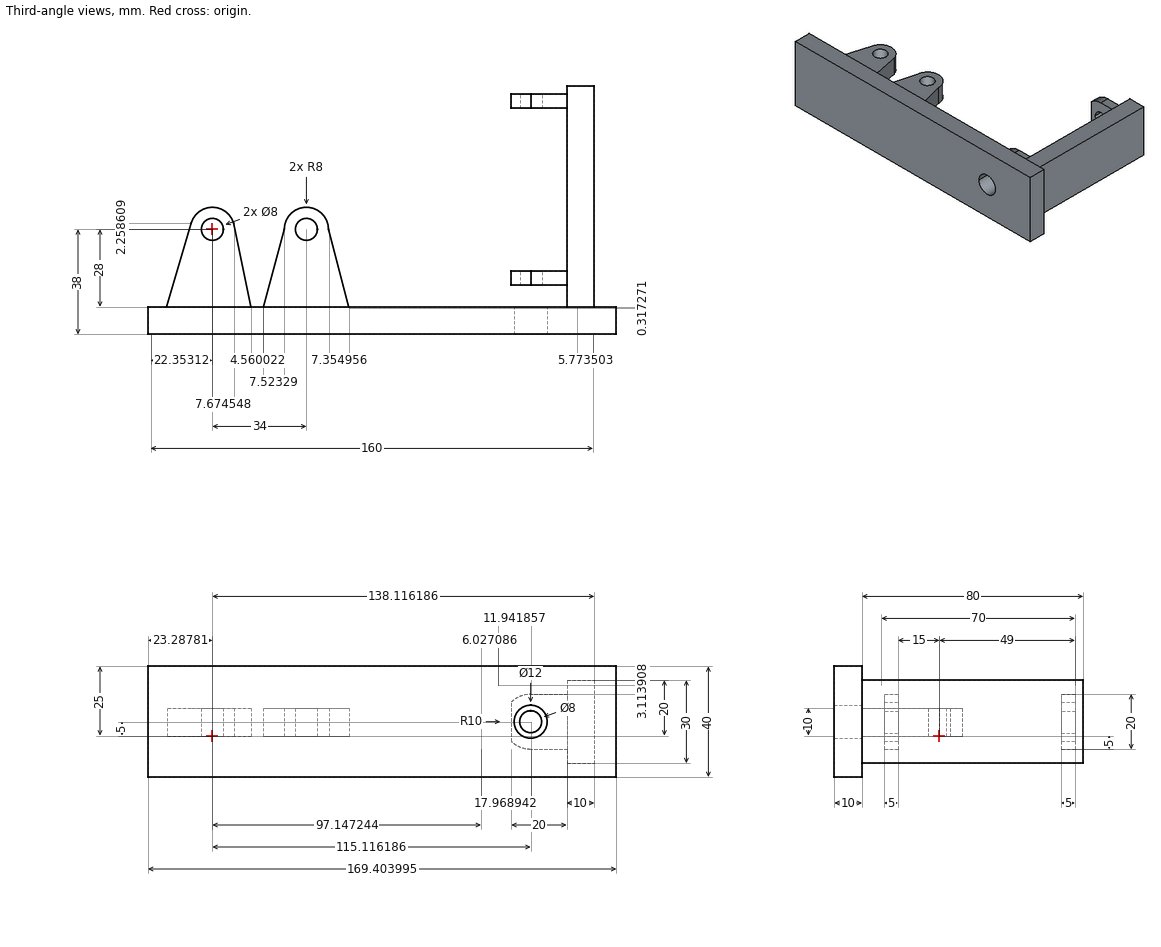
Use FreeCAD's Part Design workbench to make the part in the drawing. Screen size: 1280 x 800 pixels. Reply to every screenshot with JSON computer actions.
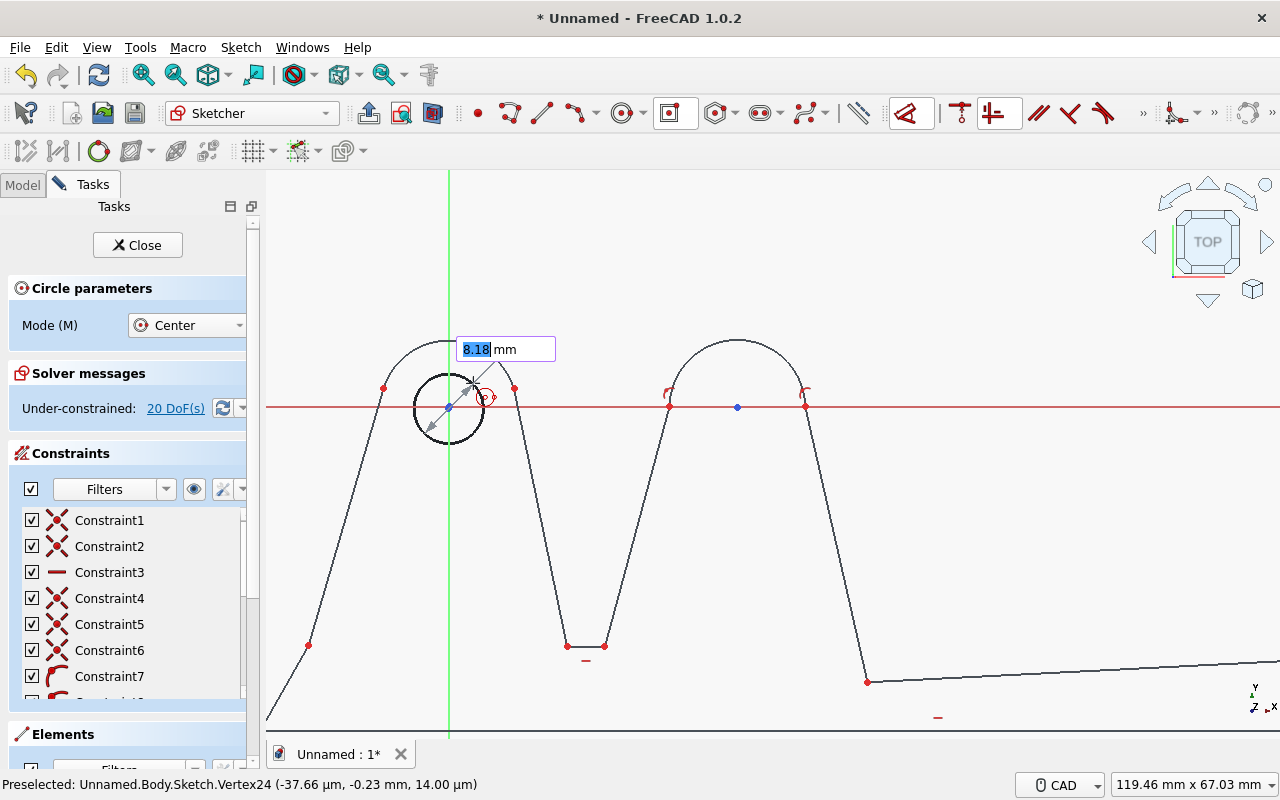
{"action": "type", "text": "8"}
{"action": "key", "text": "Return"}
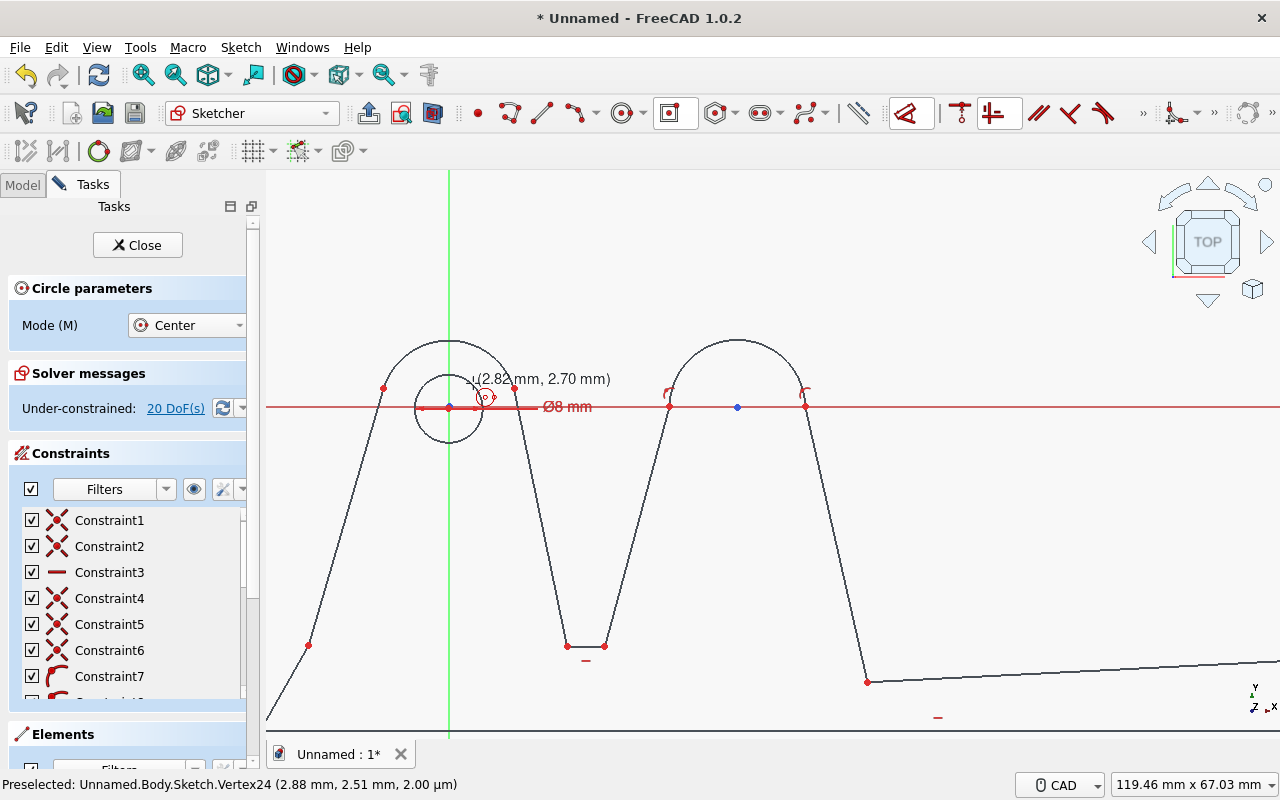
{"action": "left_click", "coordinate": [738, 407]}
{"action": "mouse_move", "coordinate": [762, 383]}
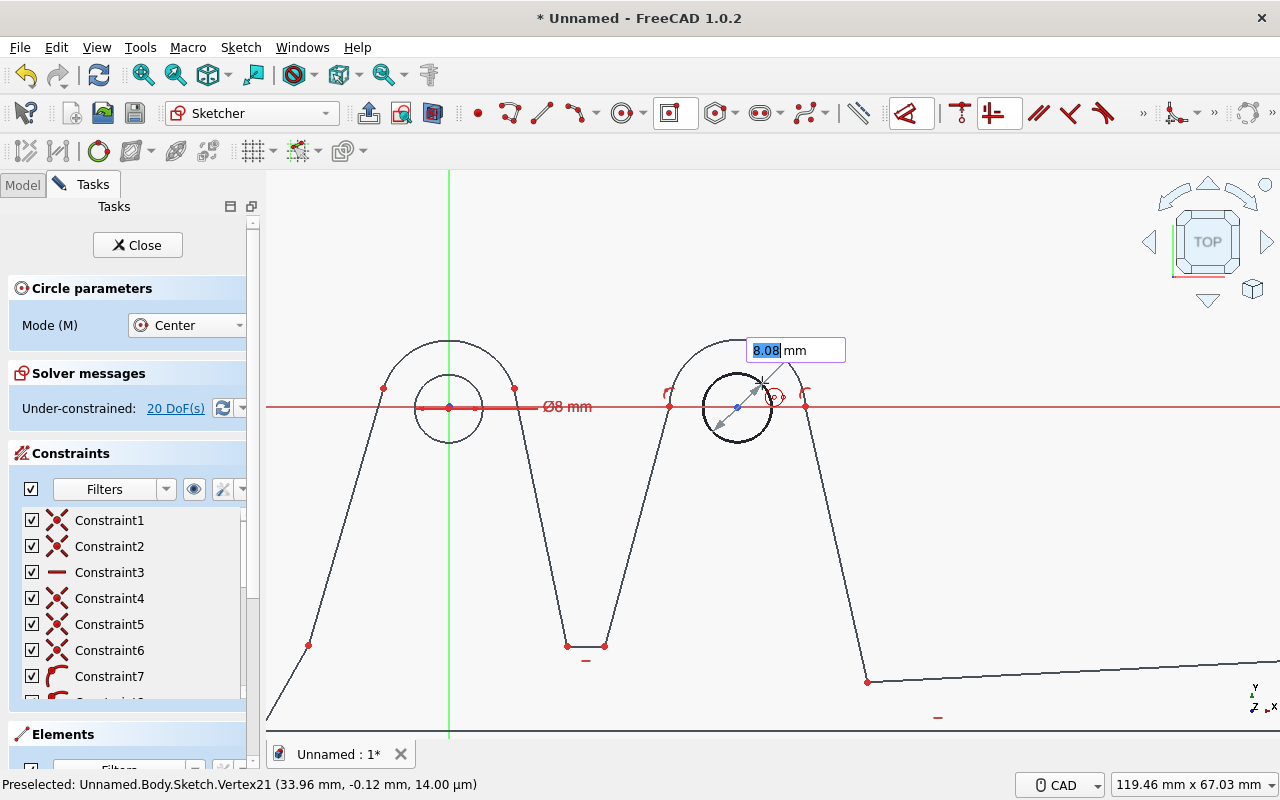
{"action": "type", "text": "8"}
{"action": "key", "text": "Return"}
{"action": "key", "text": "Escape"}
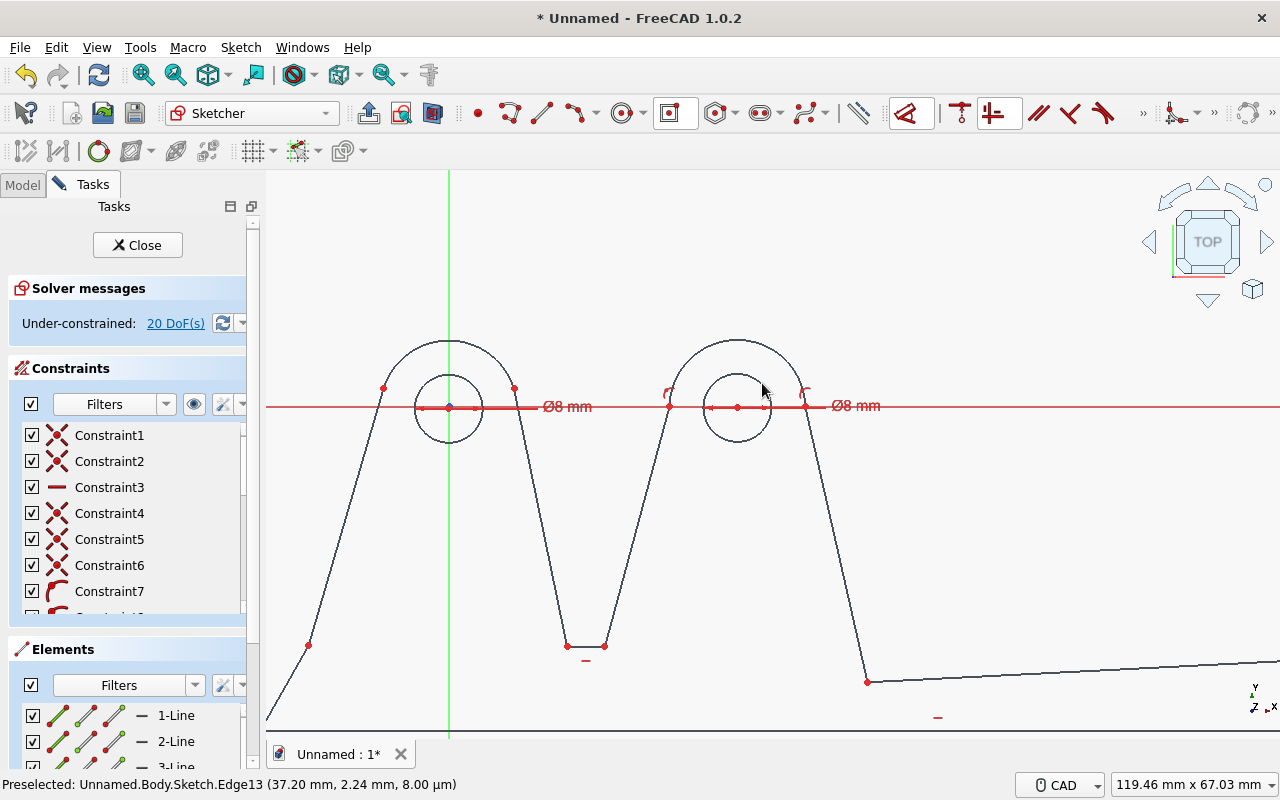
{"action": "left_click", "coordinate": [361, 466]}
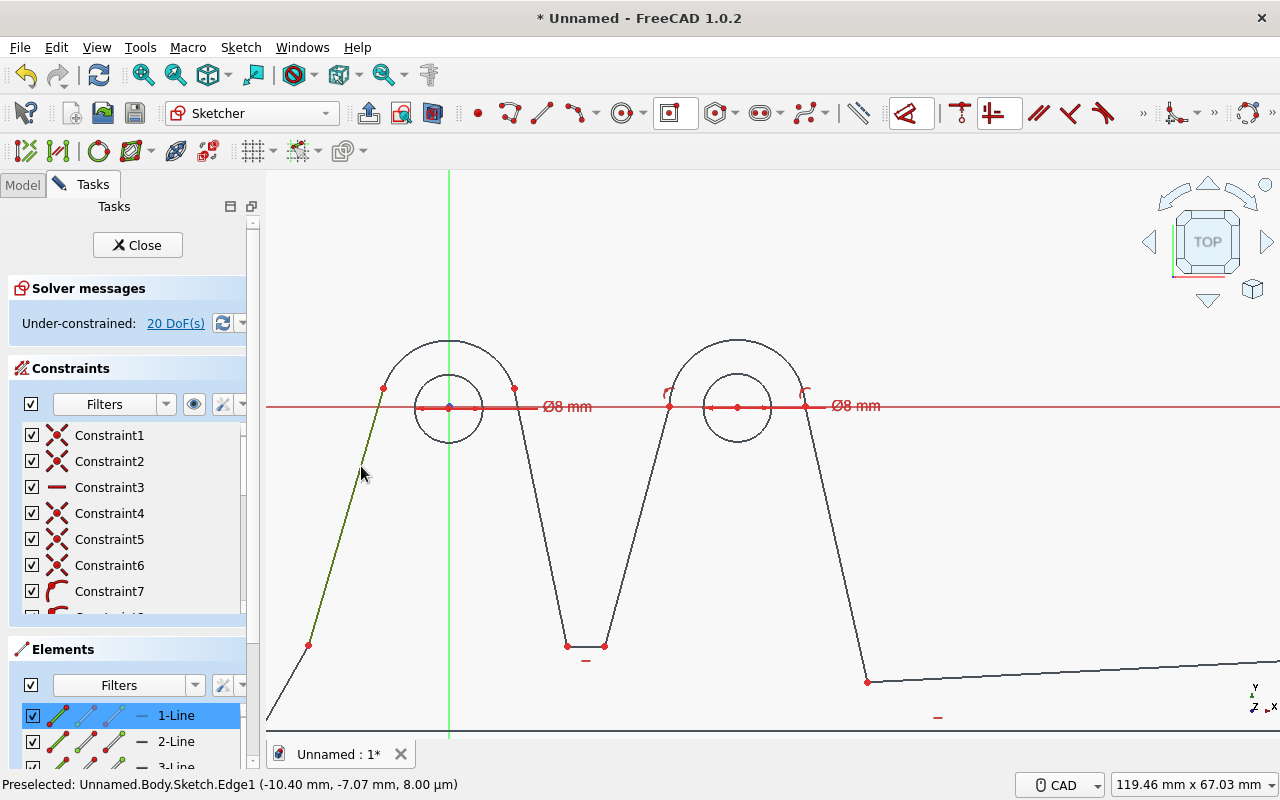
{"action": "left_click", "coordinate": [482, 349]}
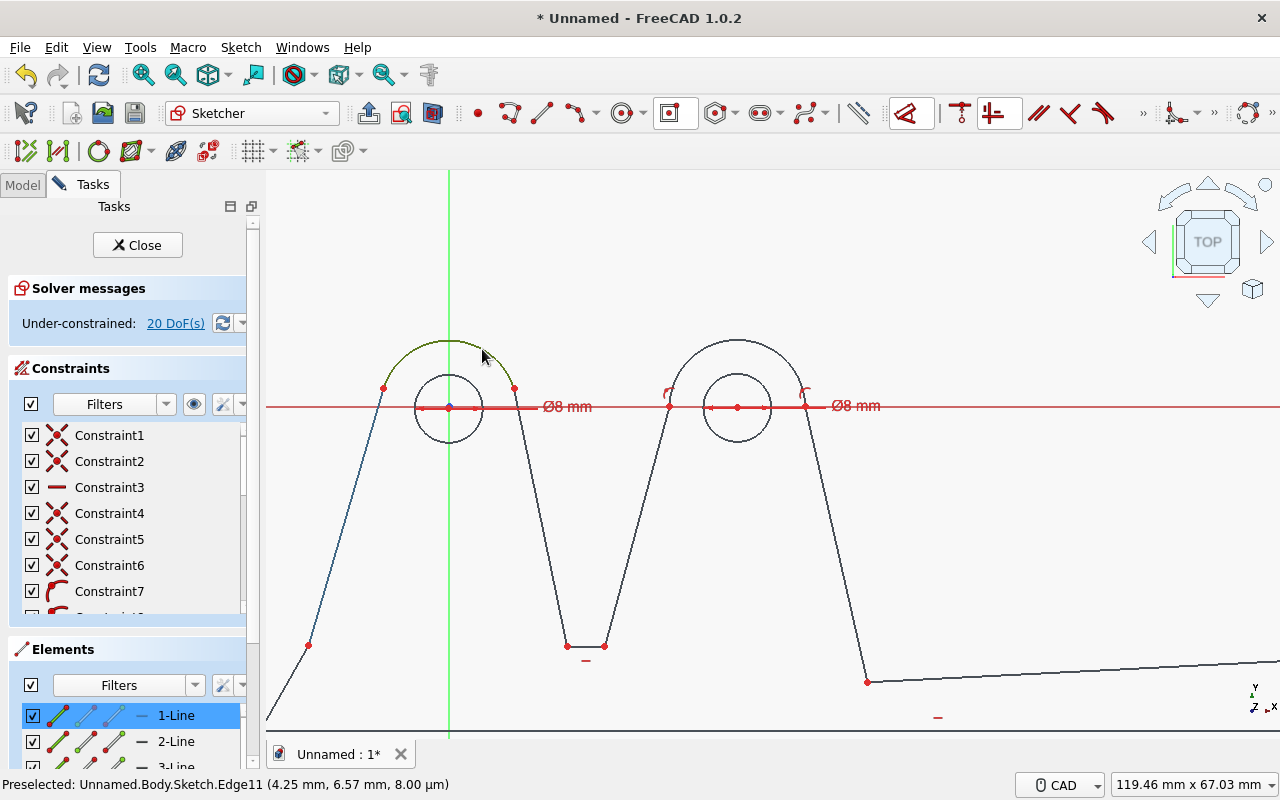
{"action": "left_click", "coordinate": [1104, 114]}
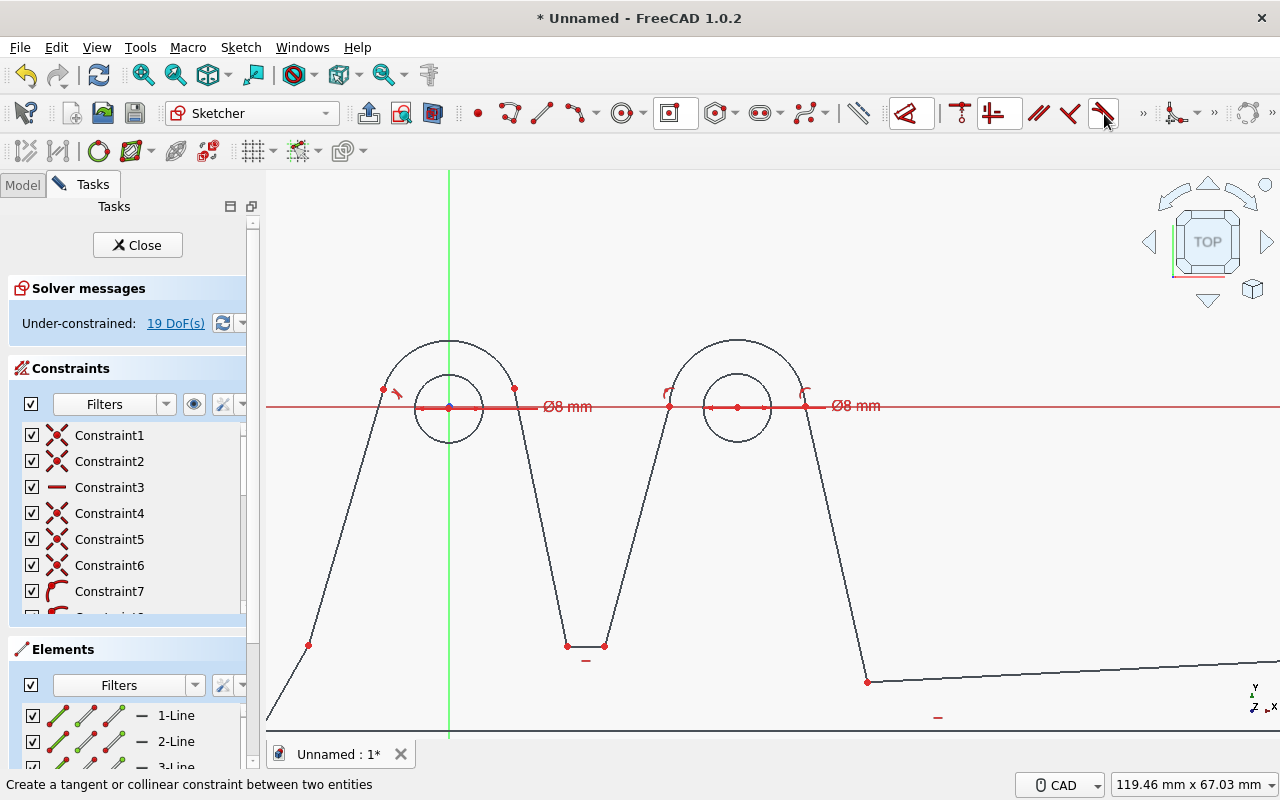
{"action": "left_click_drag", "start_coordinate": [439, 397], "coordinate": [459, 419]}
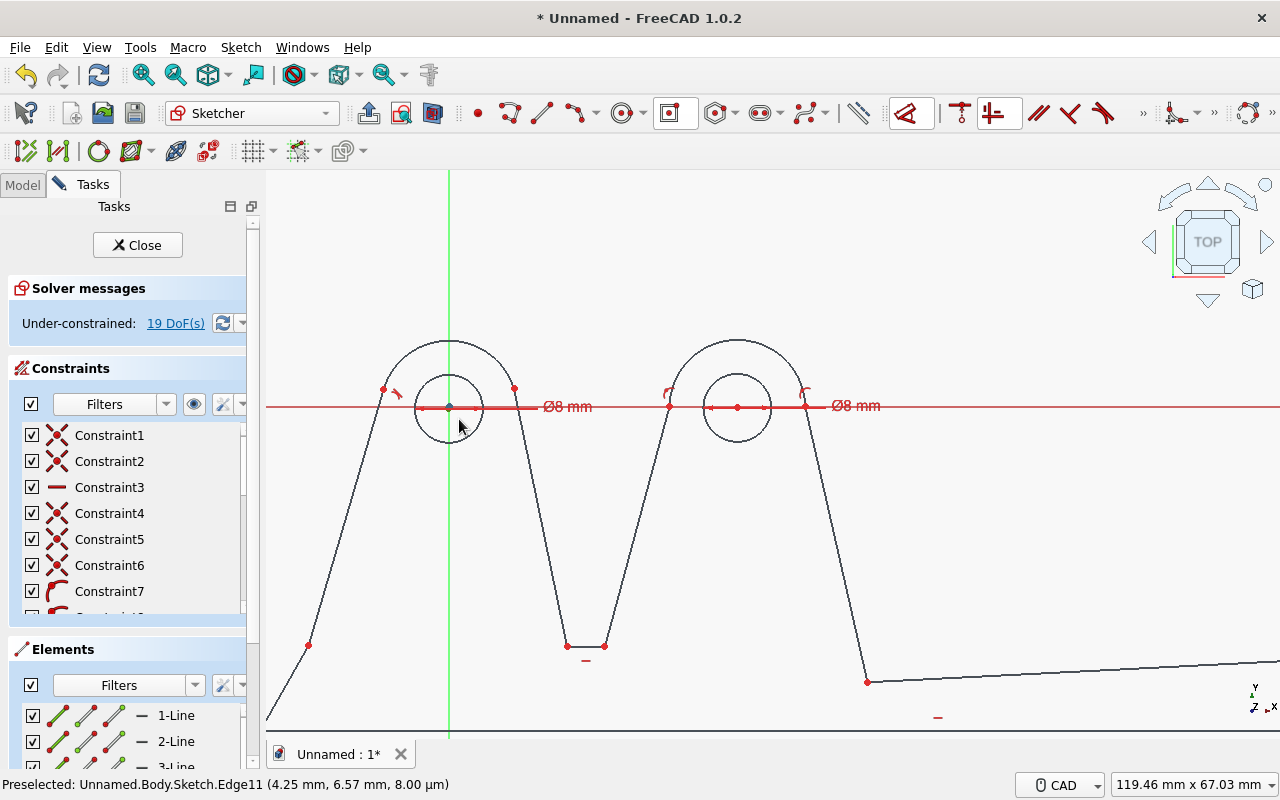
{"action": "left_click", "coordinate": [960, 114]}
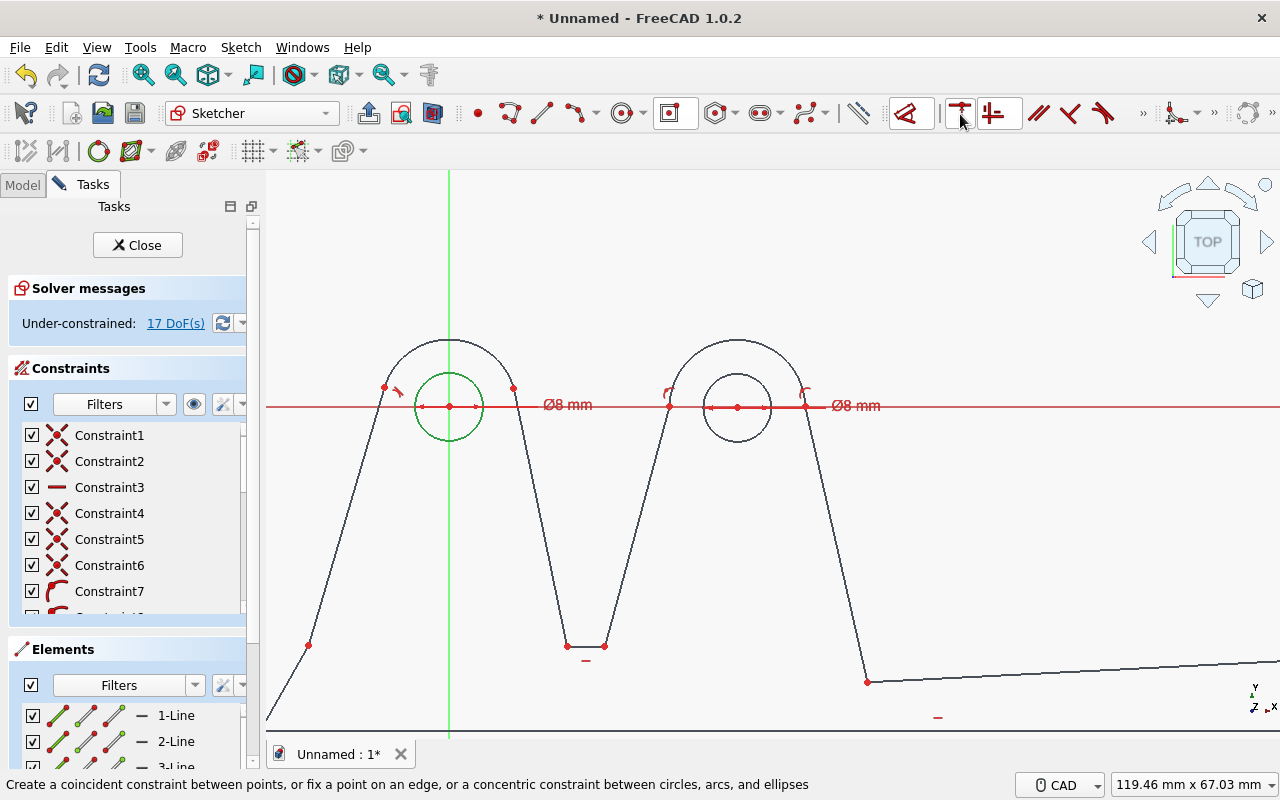
{"action": "left_click", "coordinate": [777, 353]}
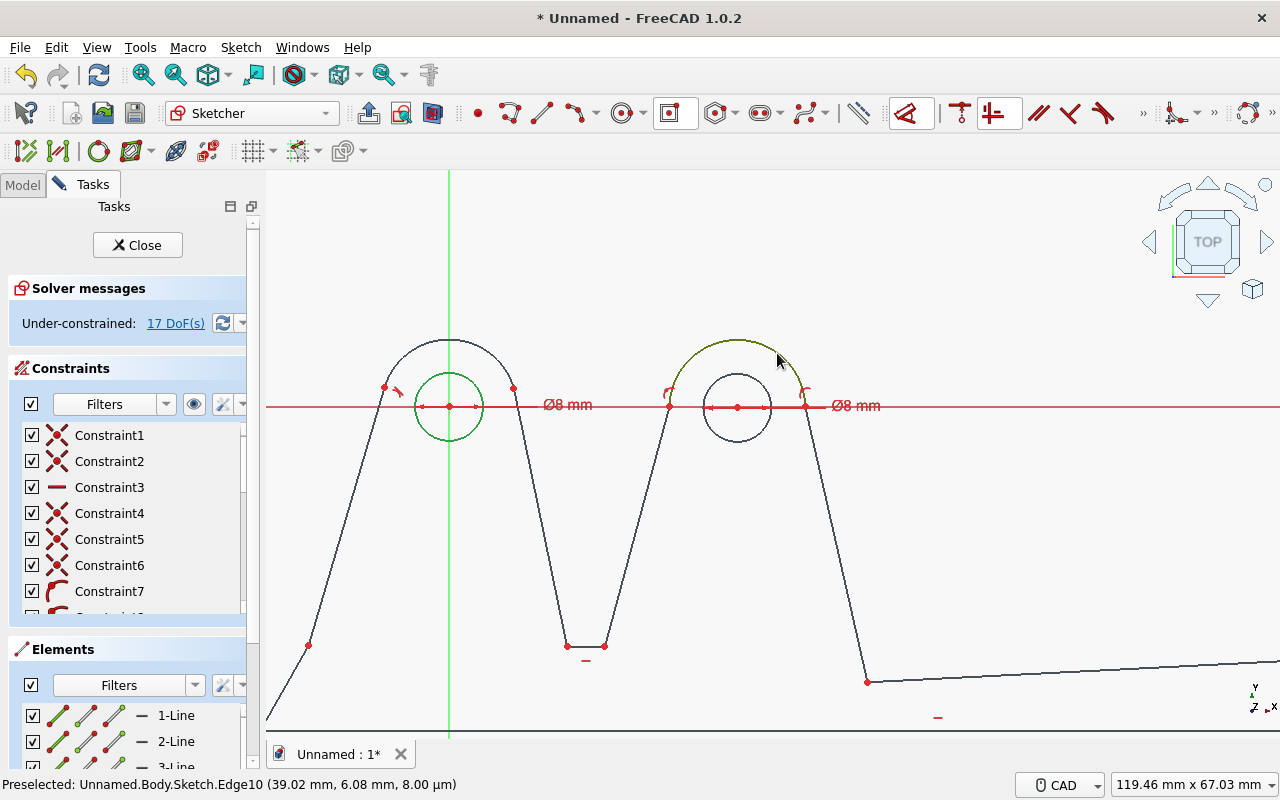
{"action": "left_click", "coordinate": [483, 349]}